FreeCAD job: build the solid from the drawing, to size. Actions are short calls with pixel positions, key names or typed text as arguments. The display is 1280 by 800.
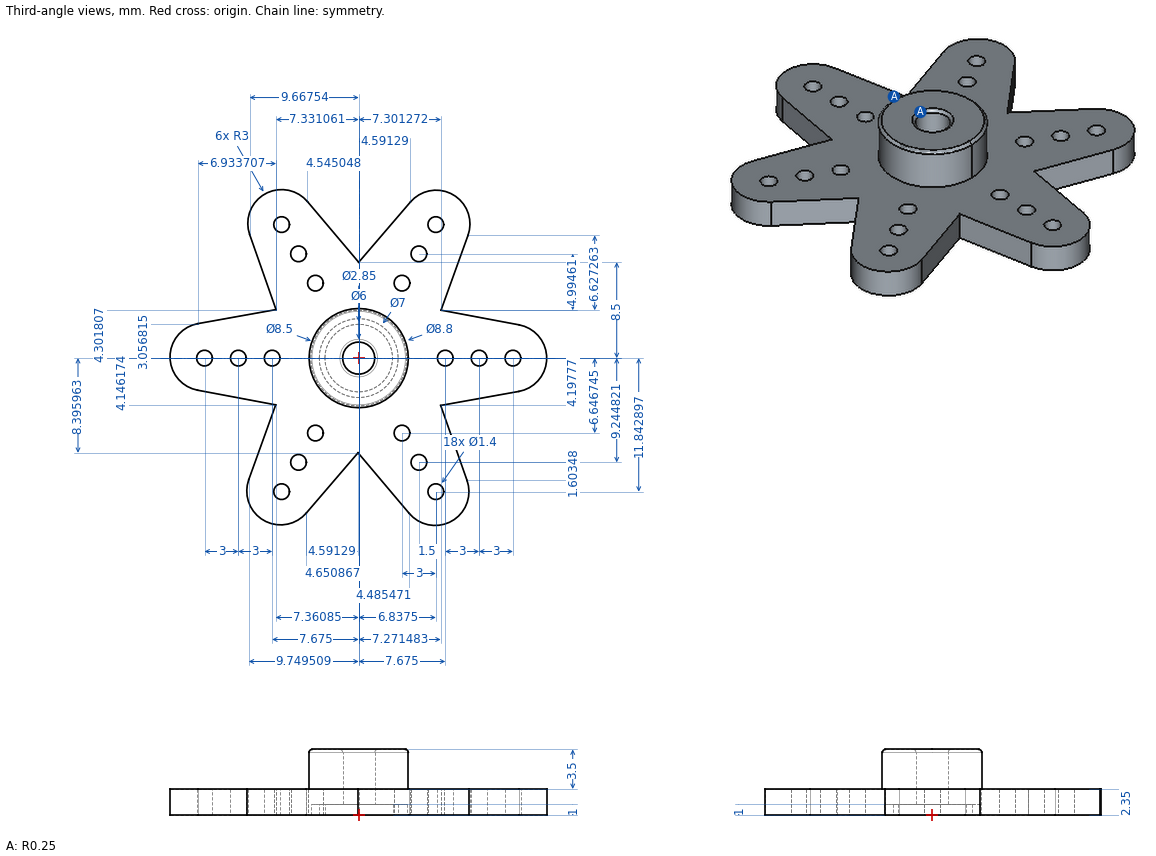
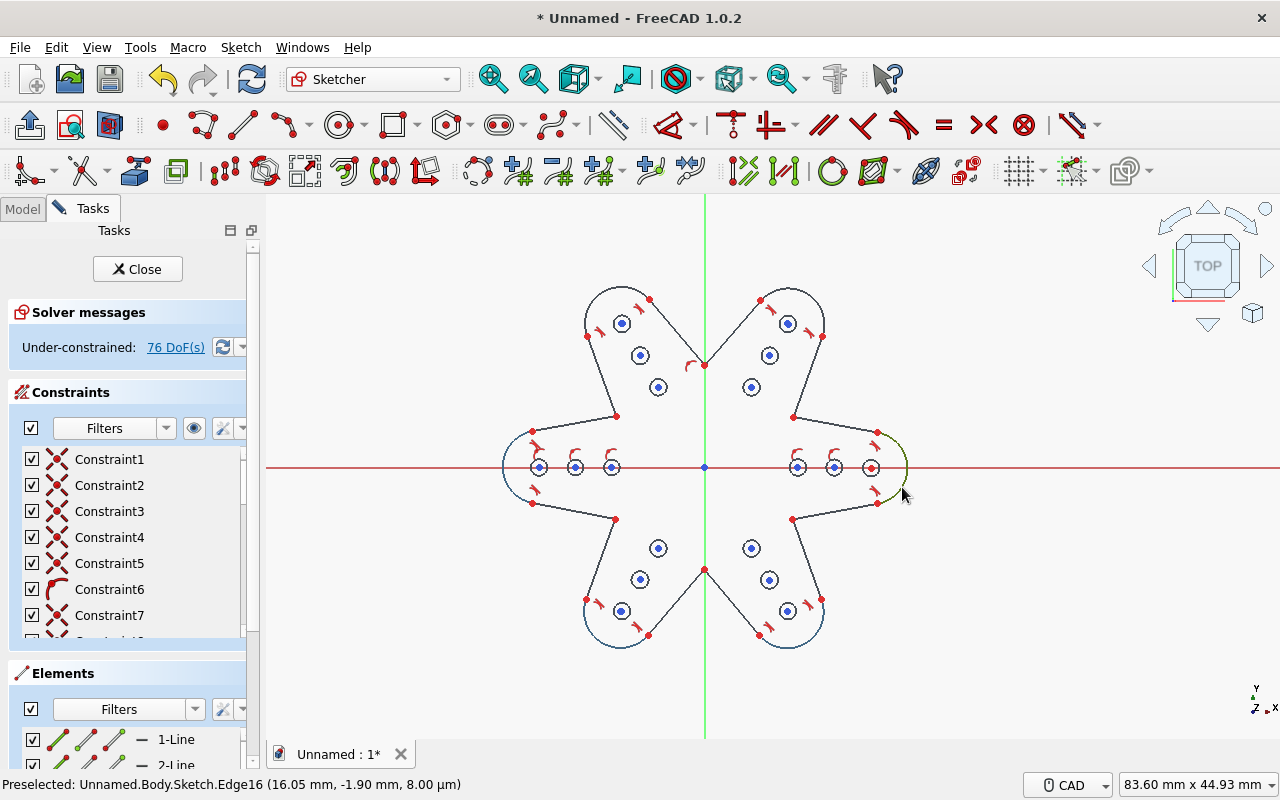
click(820, 308)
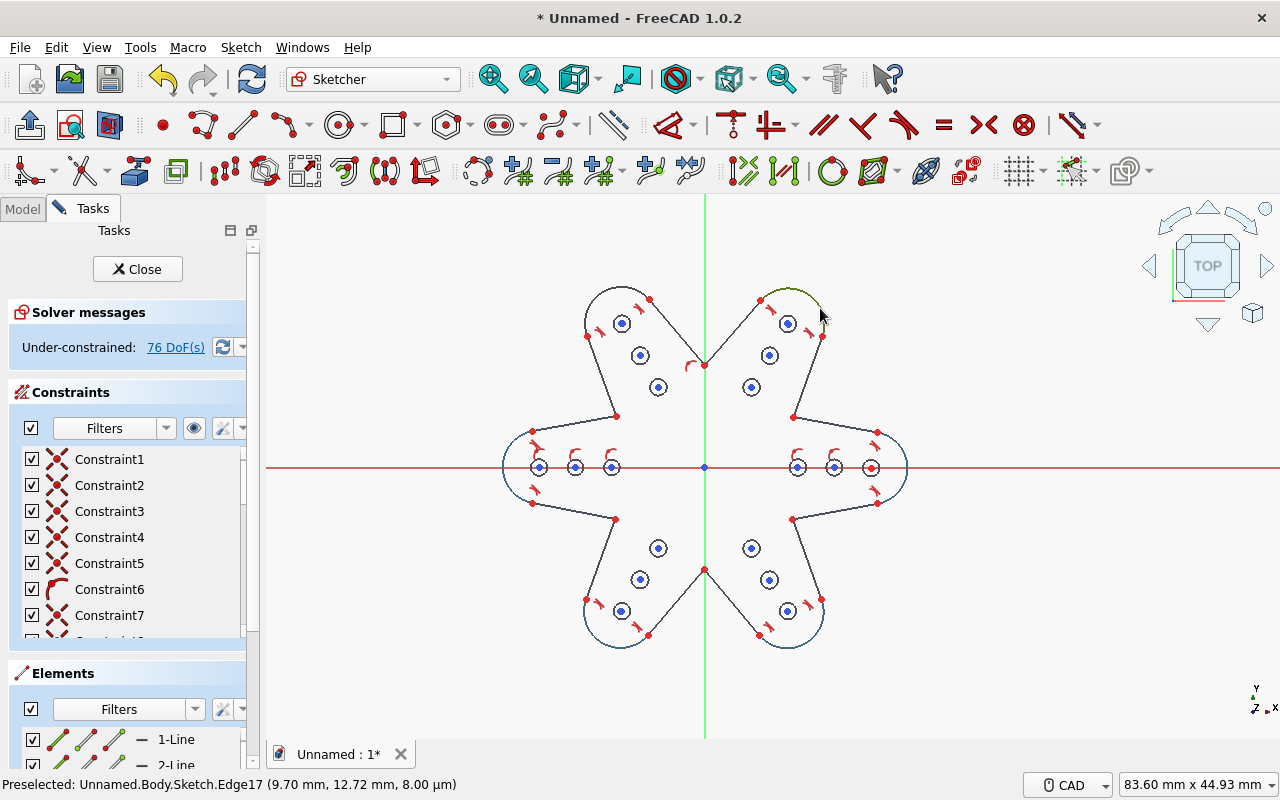
click(623, 287)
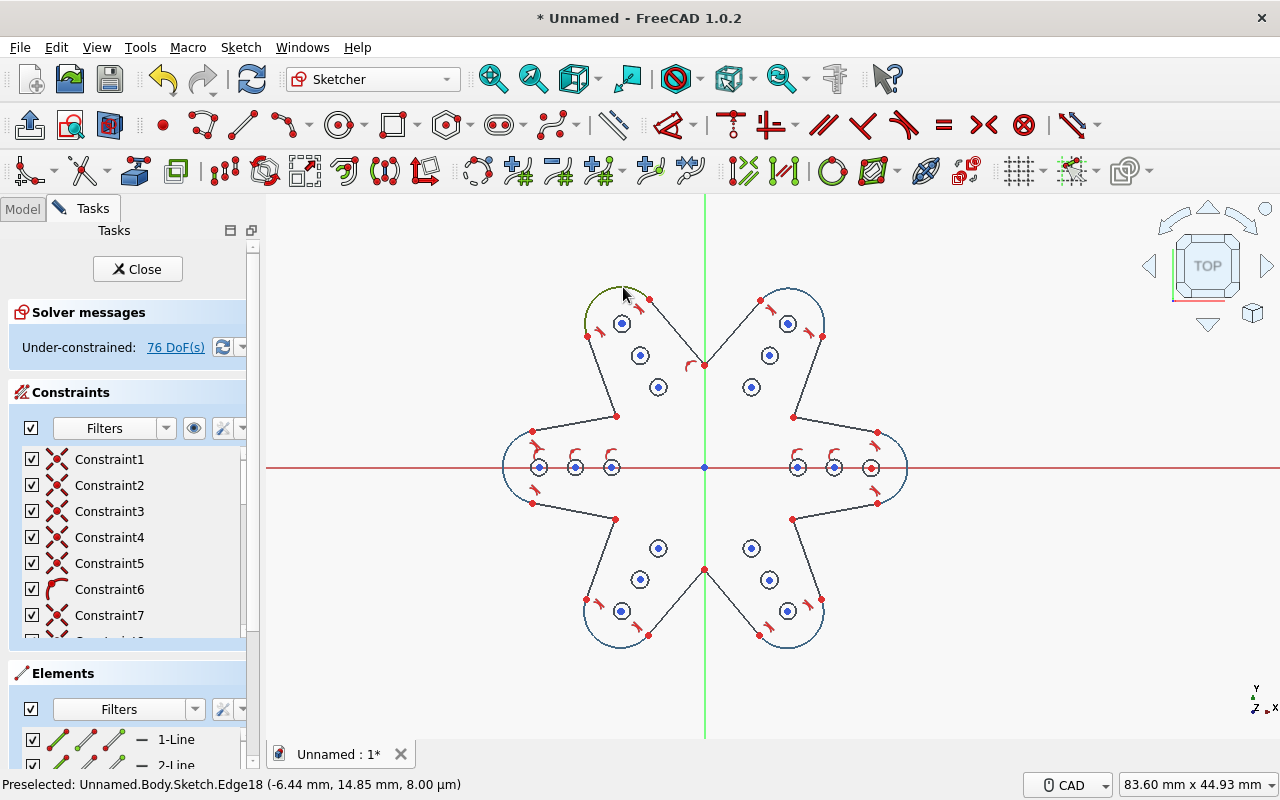
click(944, 126)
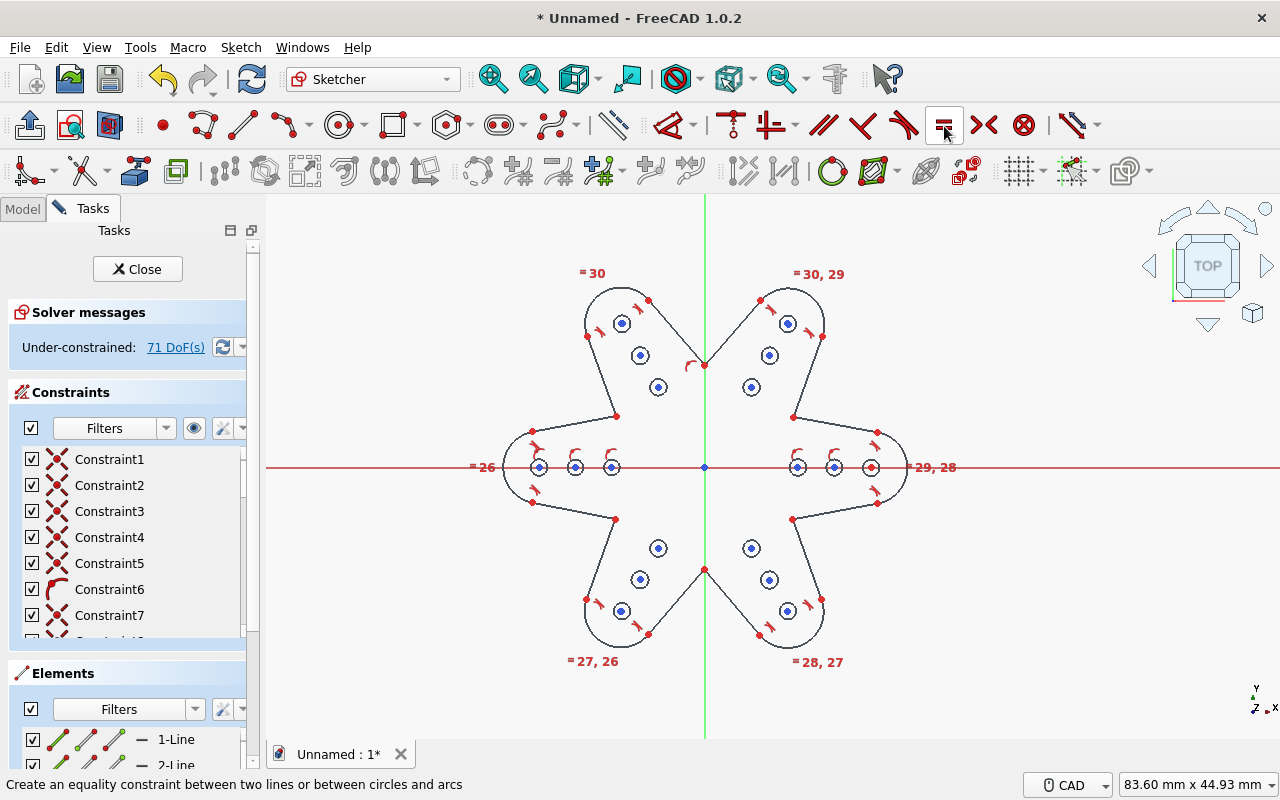
scroll(782, 617, up, 3)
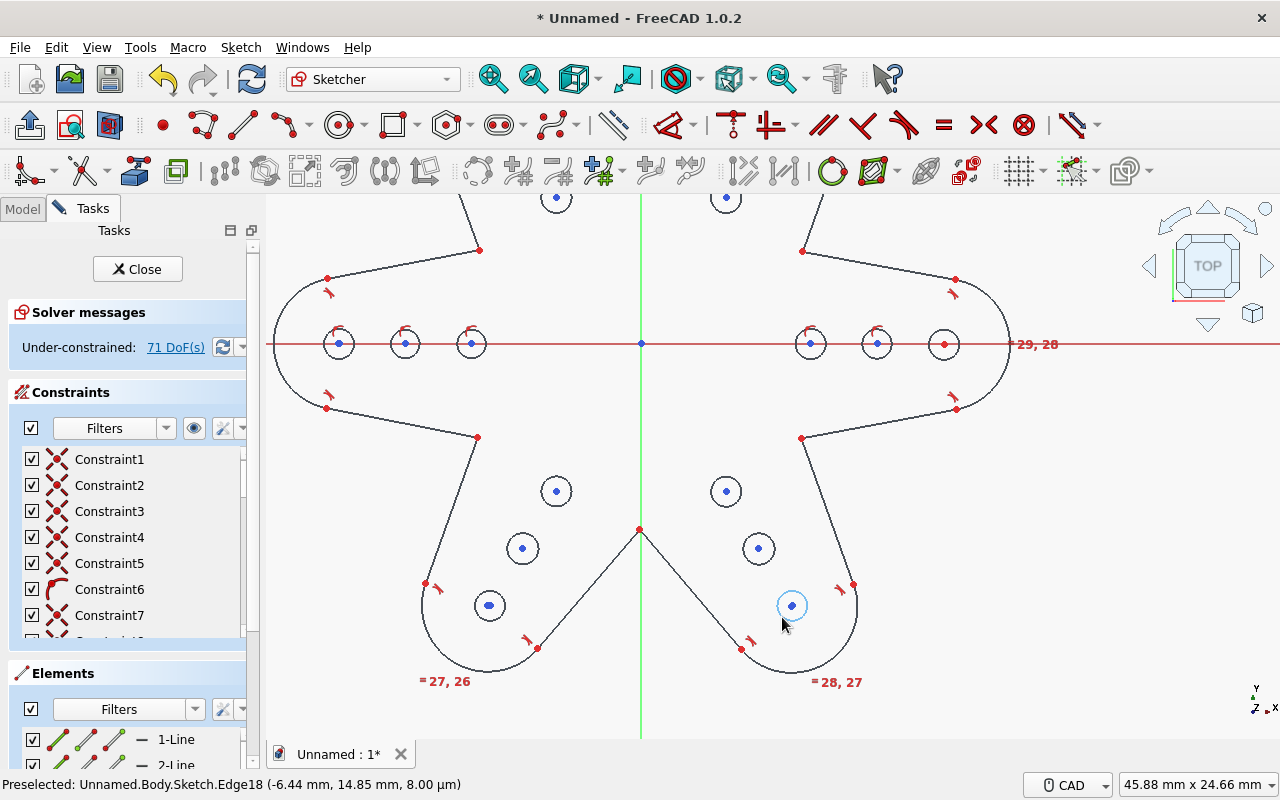
click(782, 616)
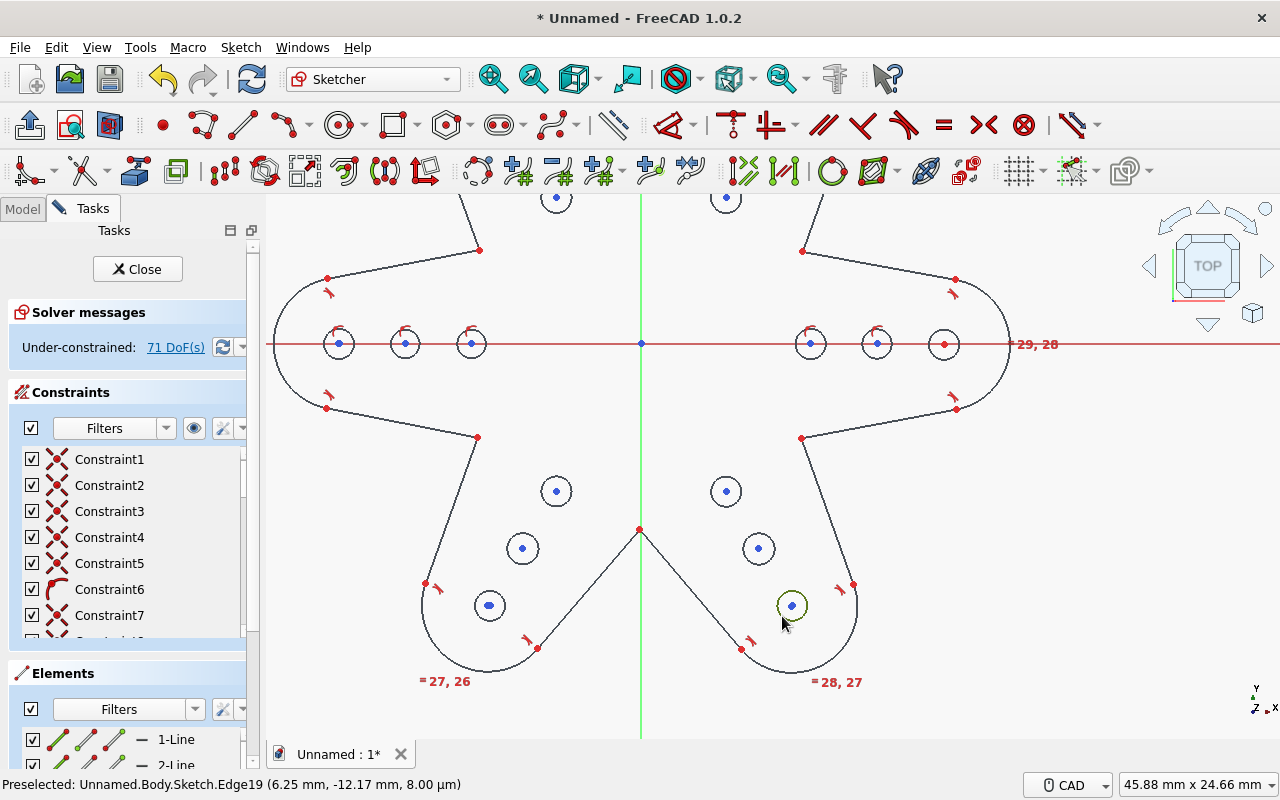
click(770, 538)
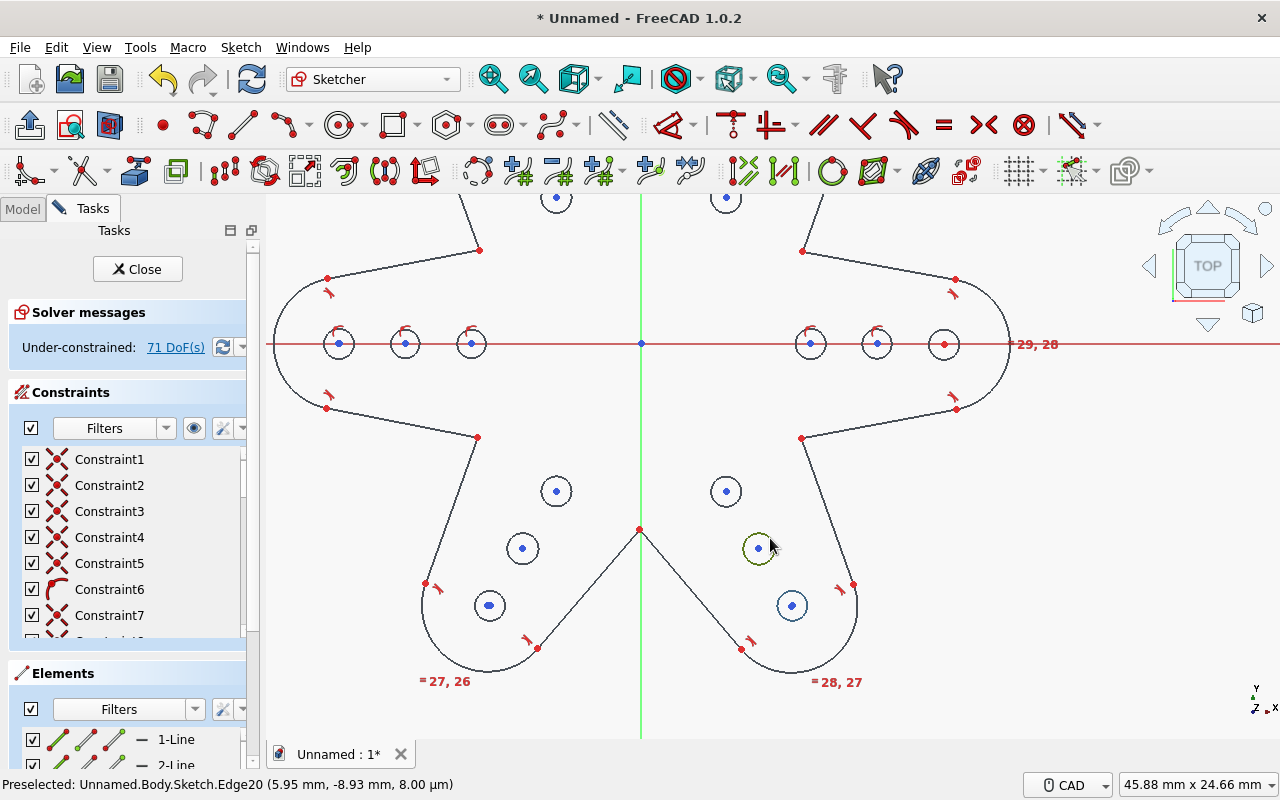
click(737, 481)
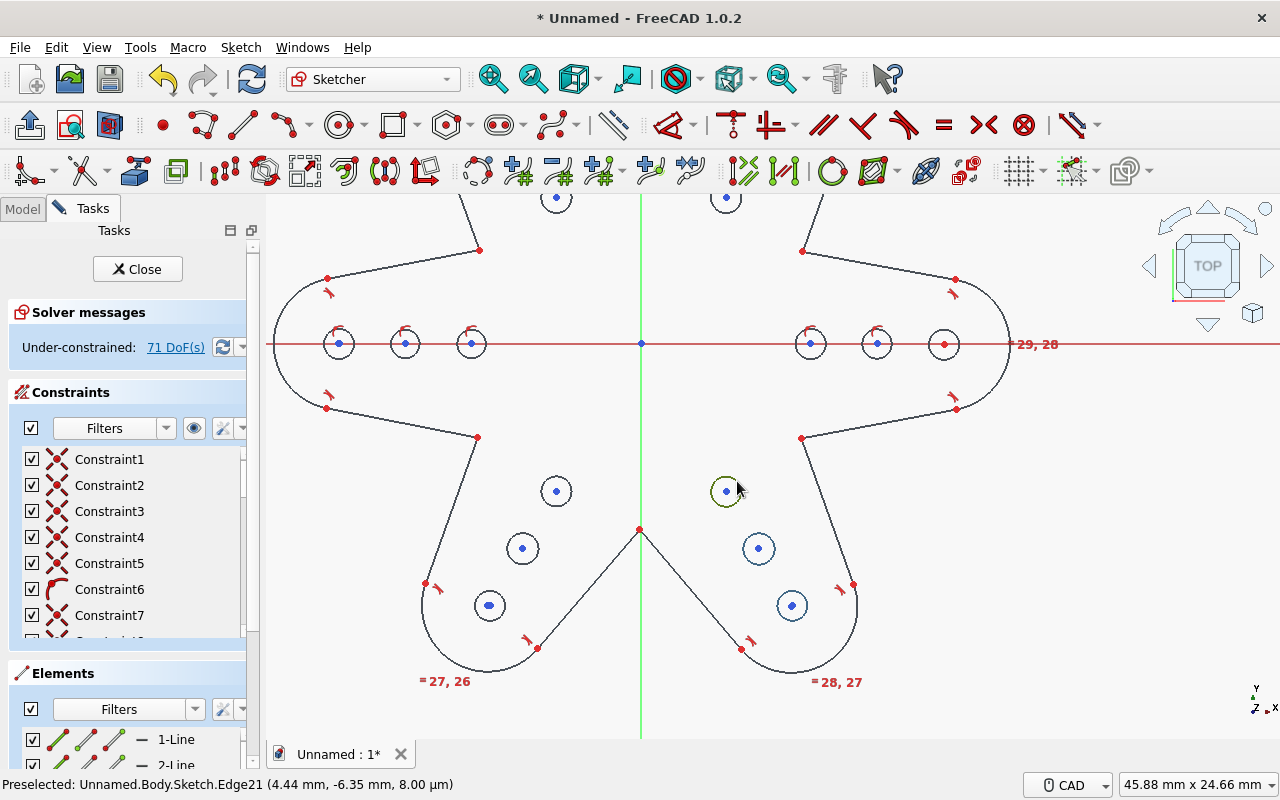
click(501, 595)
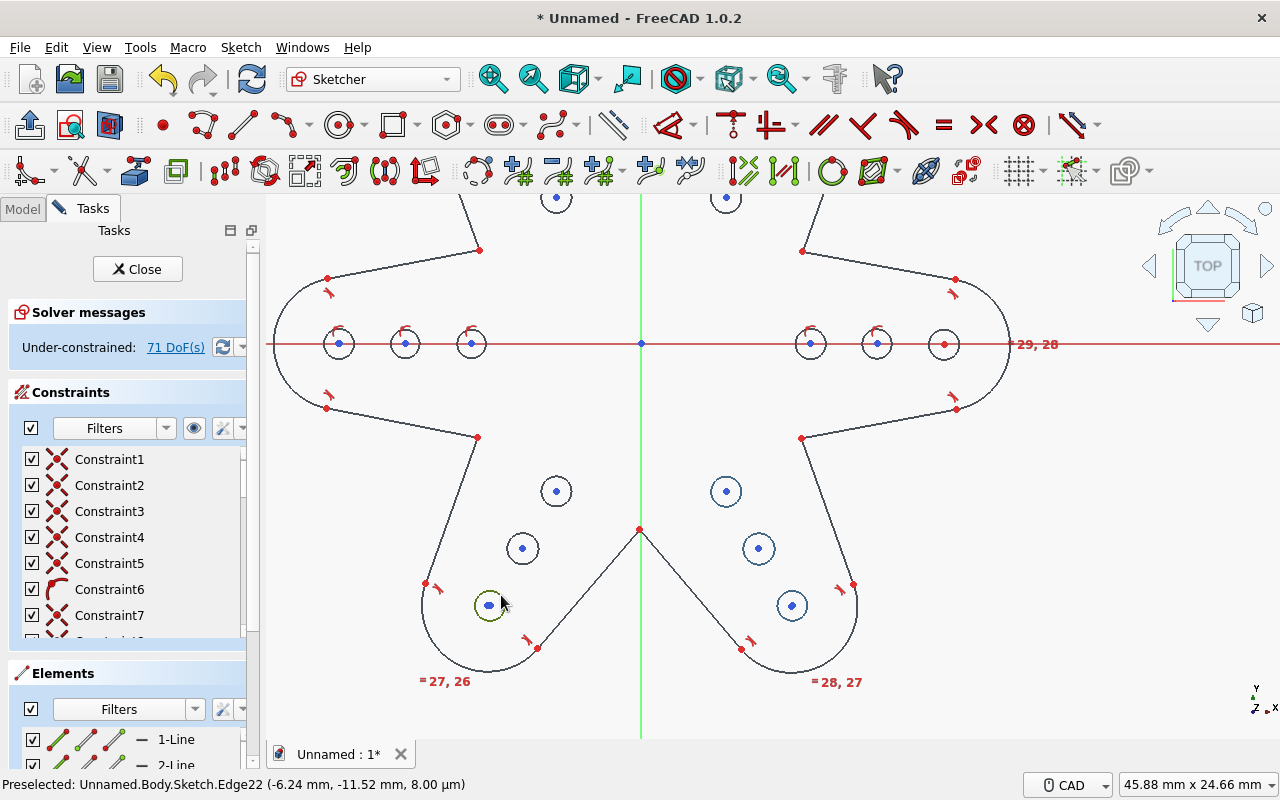
click(534, 538)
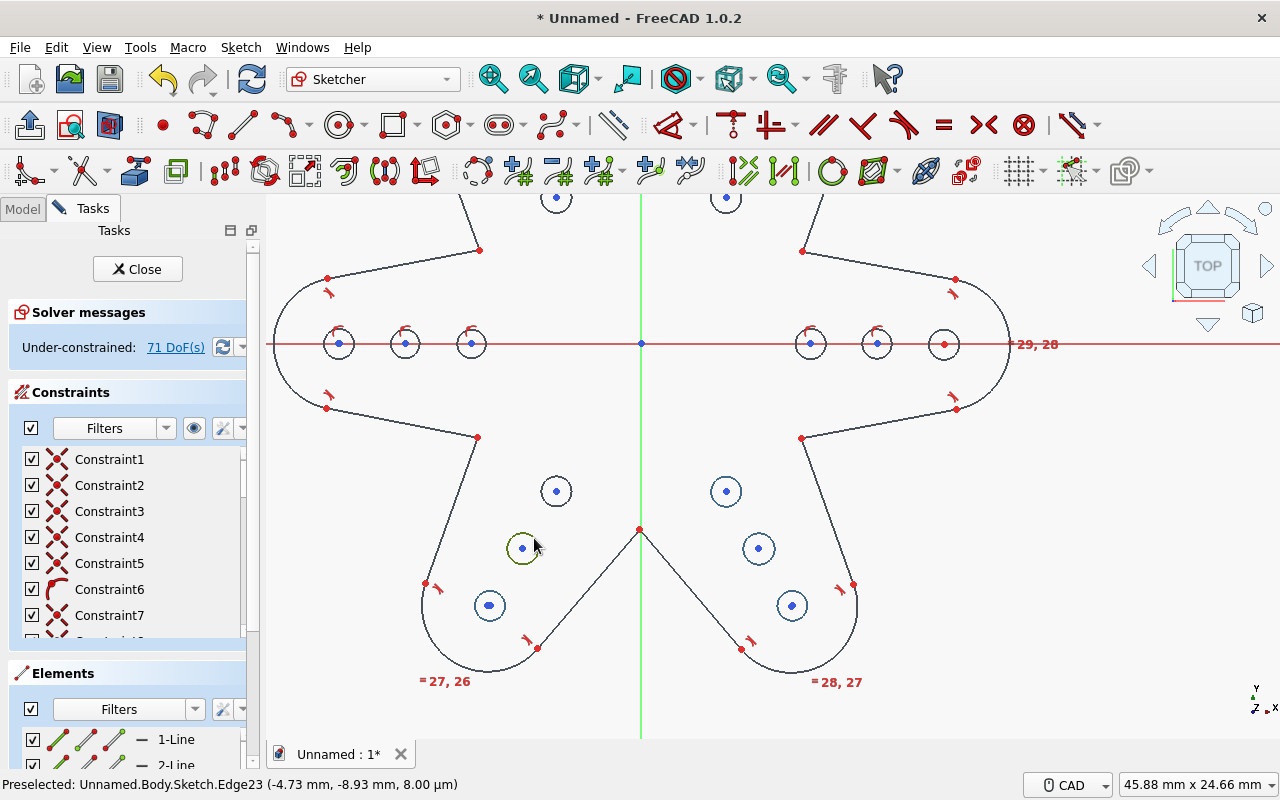
click(567, 481)